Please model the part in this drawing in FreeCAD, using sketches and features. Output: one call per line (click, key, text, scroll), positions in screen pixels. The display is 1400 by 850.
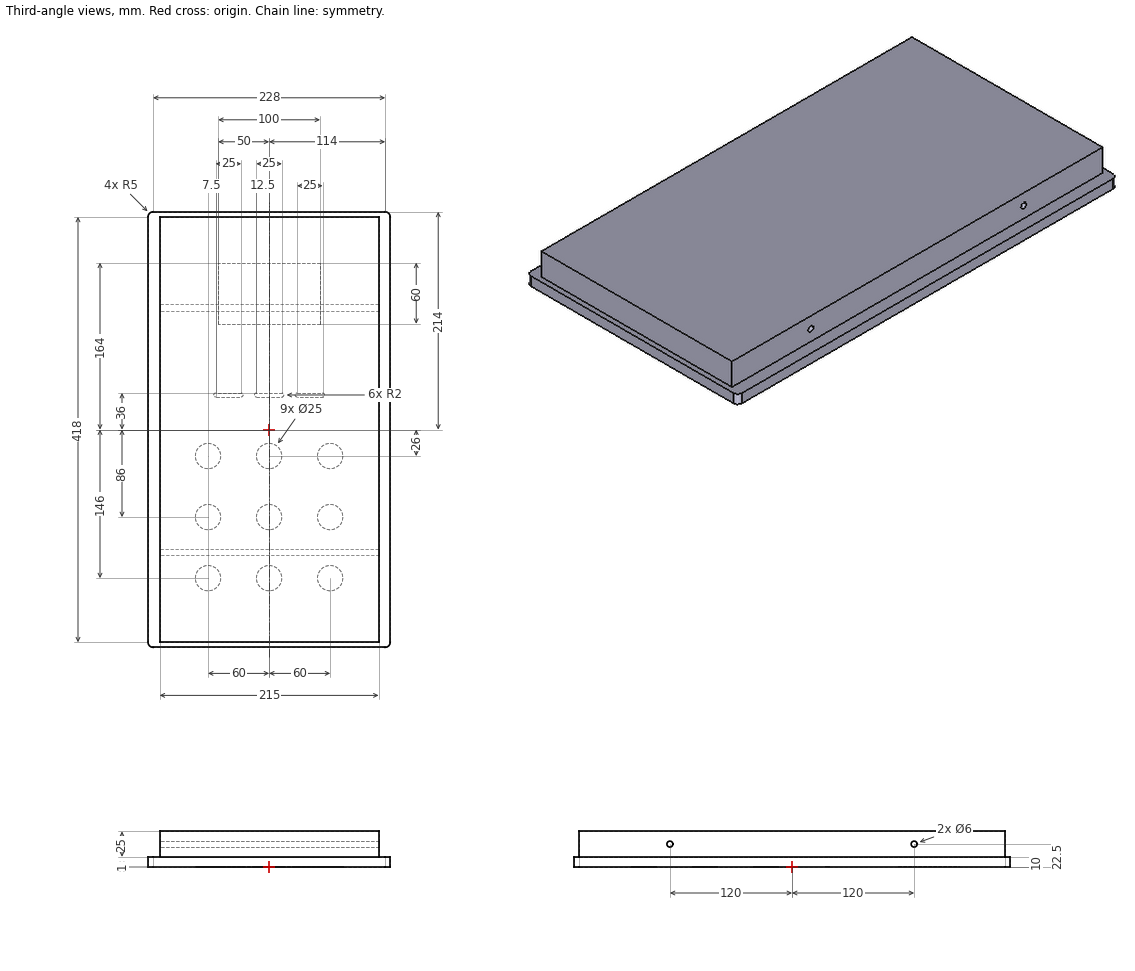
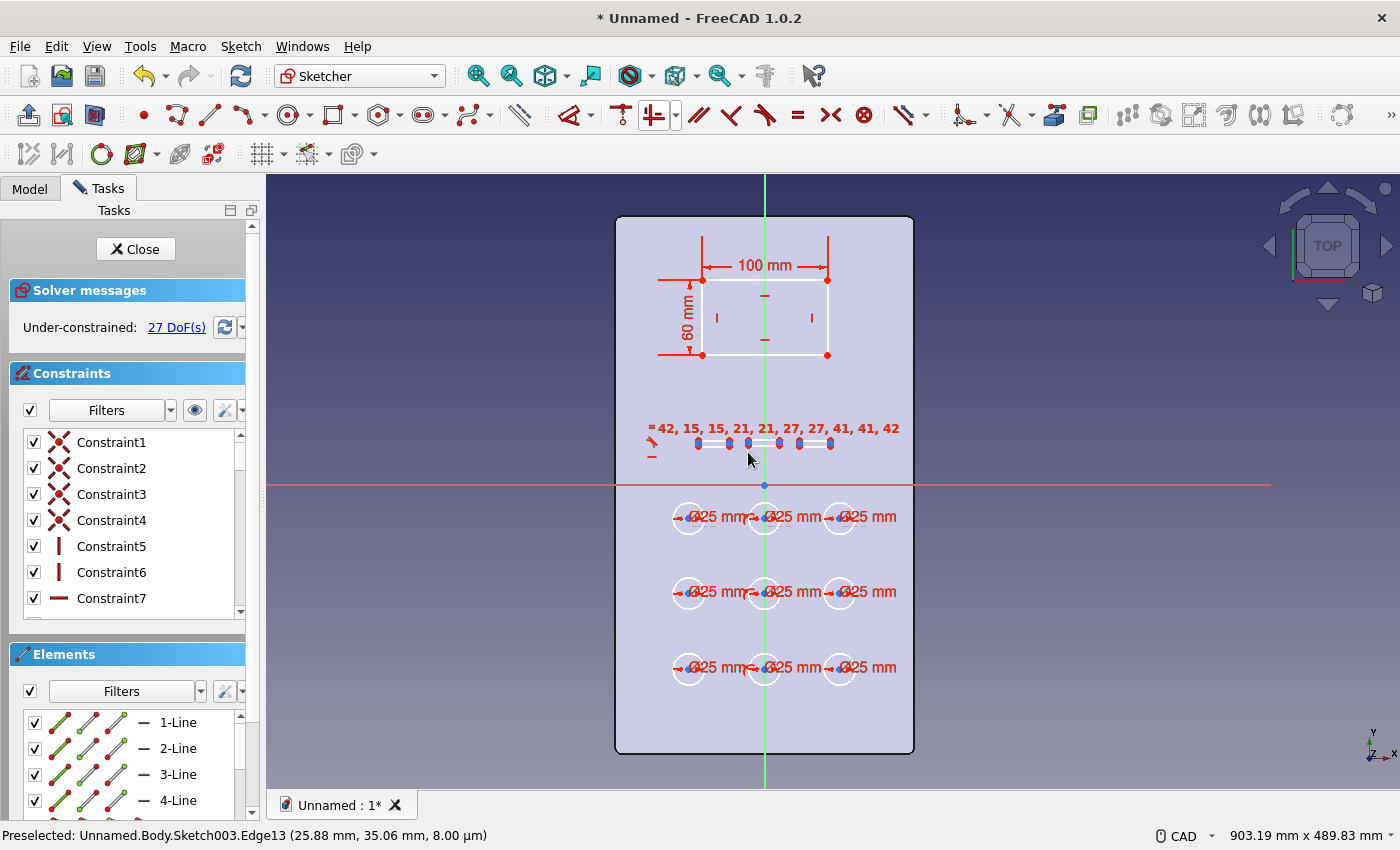
click(765, 519)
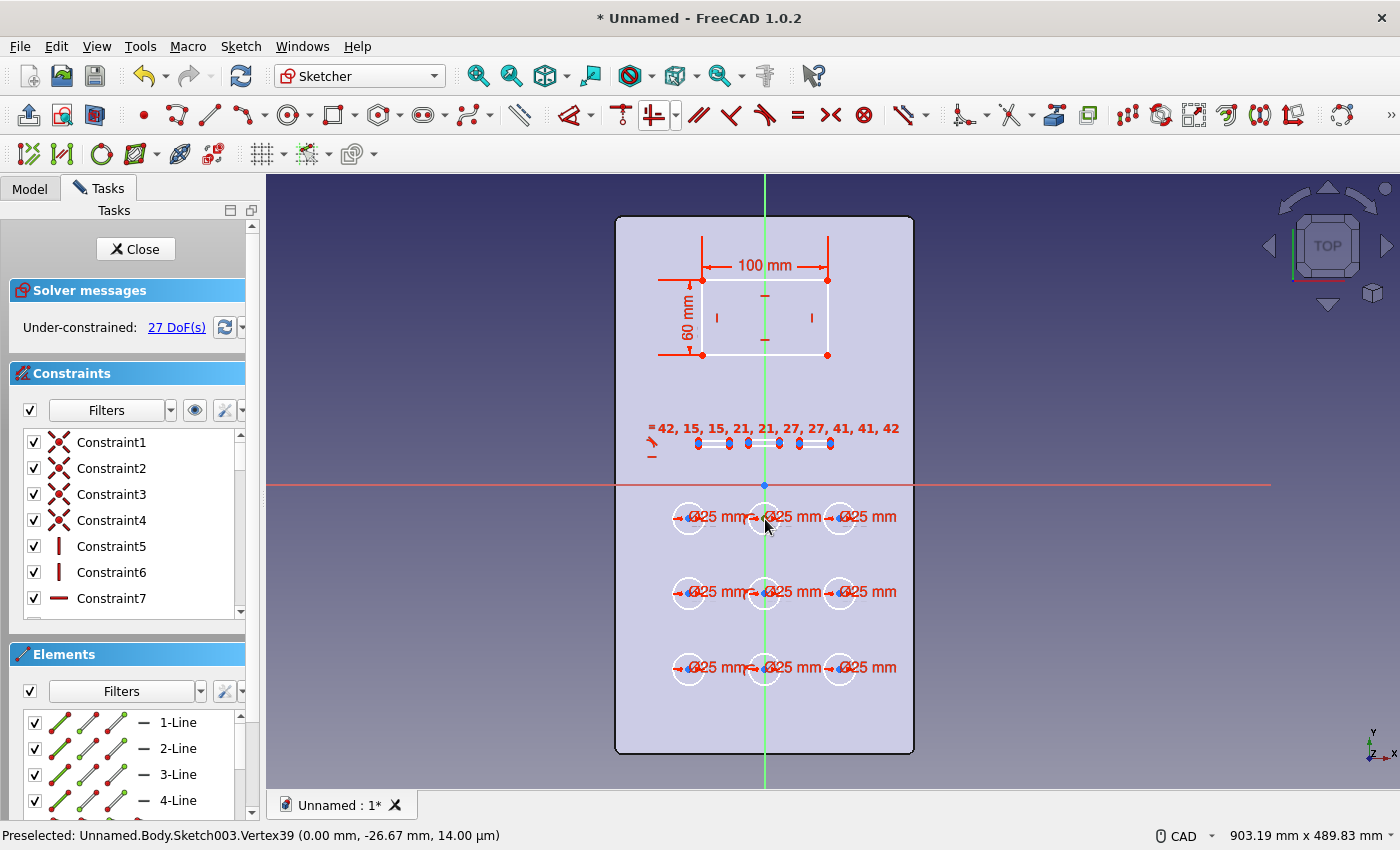
click(689, 519)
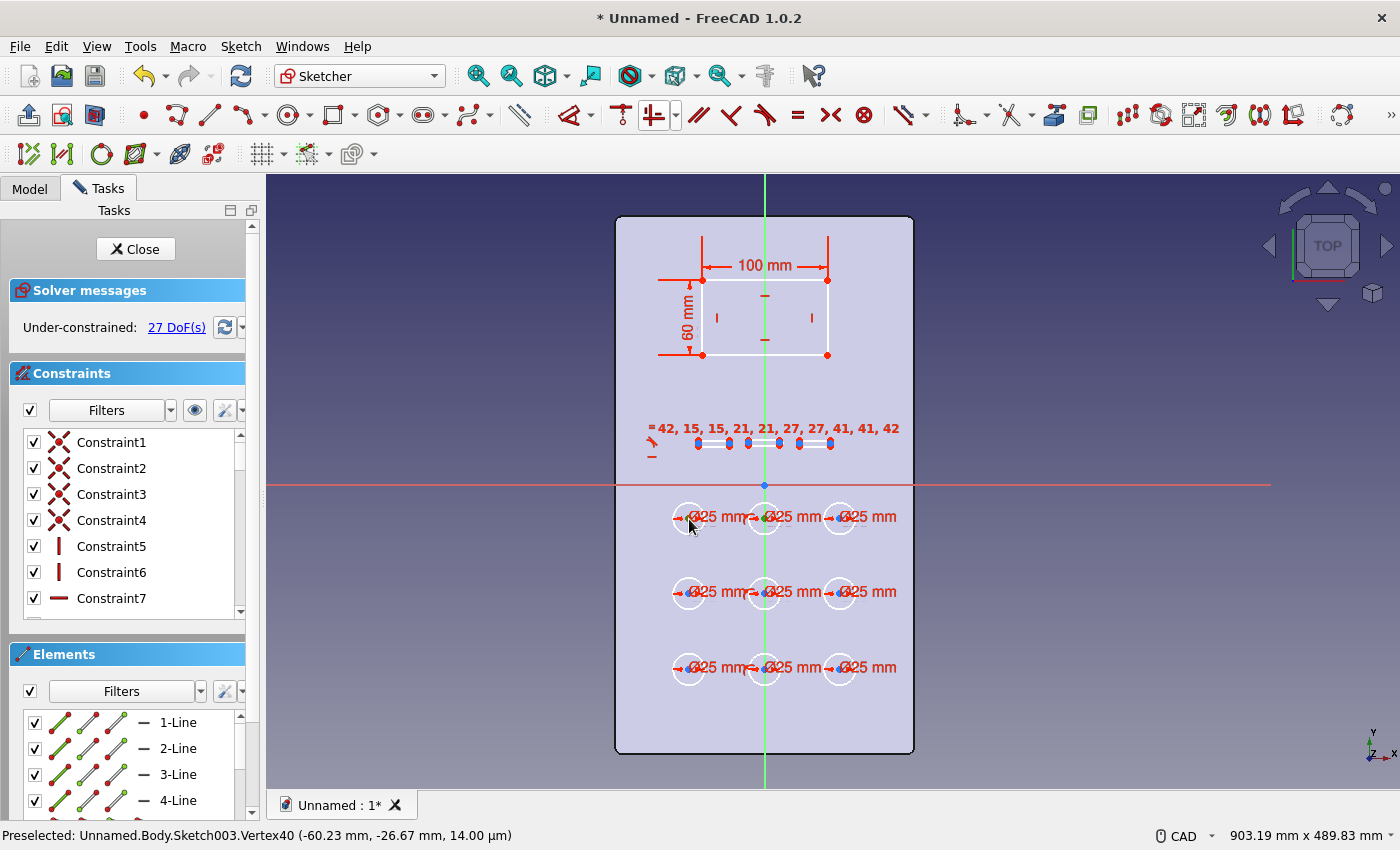
click(676, 116)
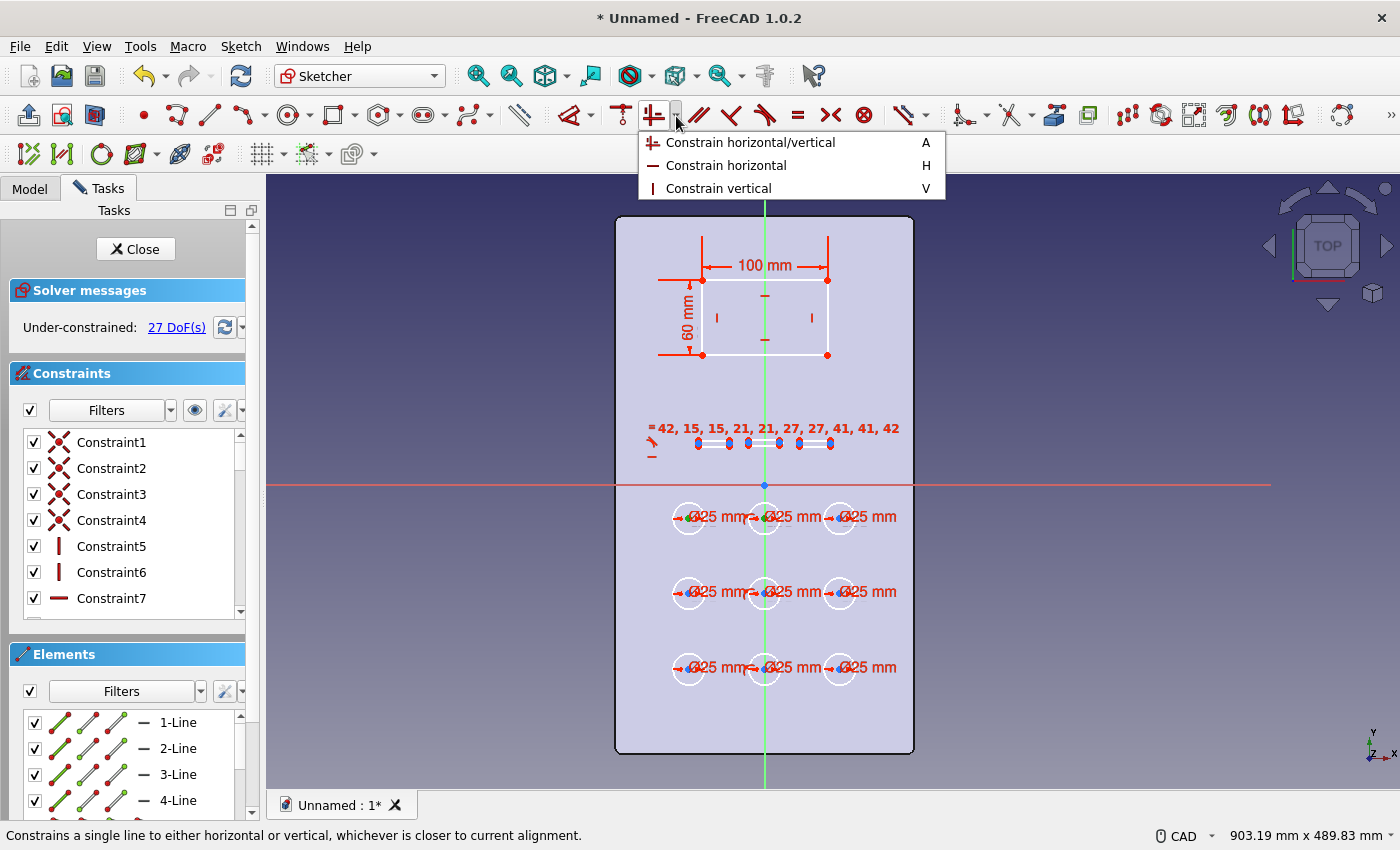
click(792, 166)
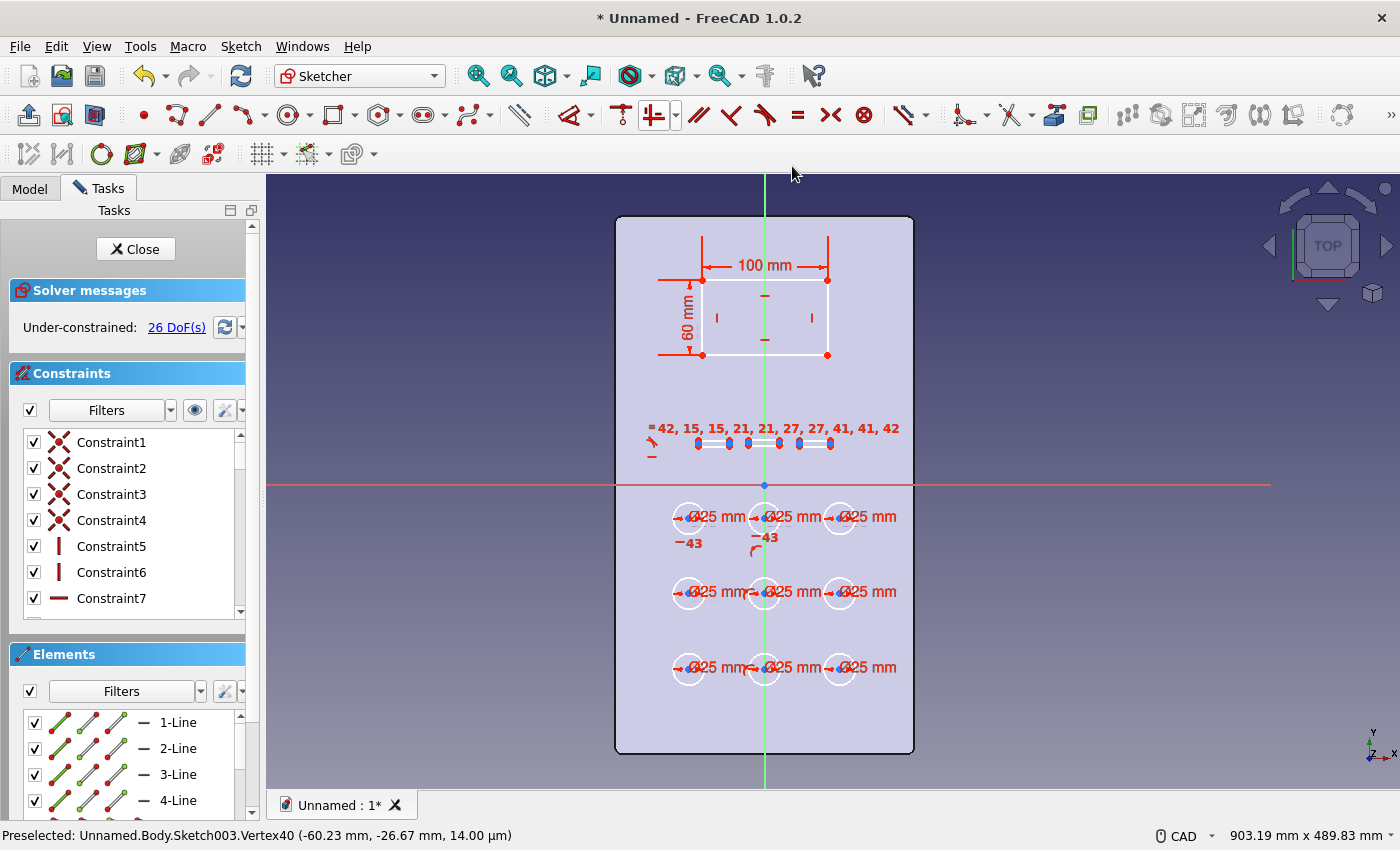
click(689, 519)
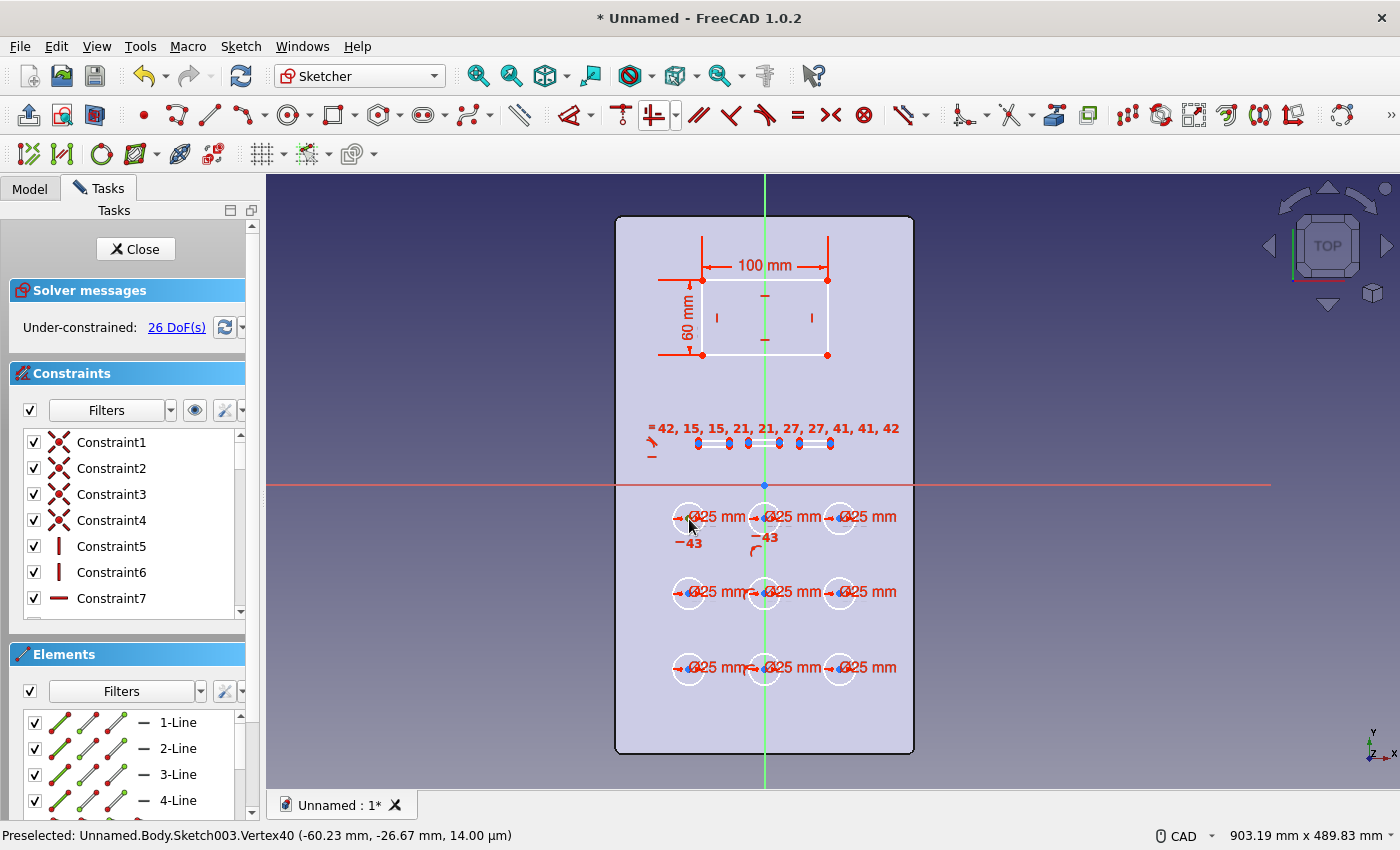
click(689, 594)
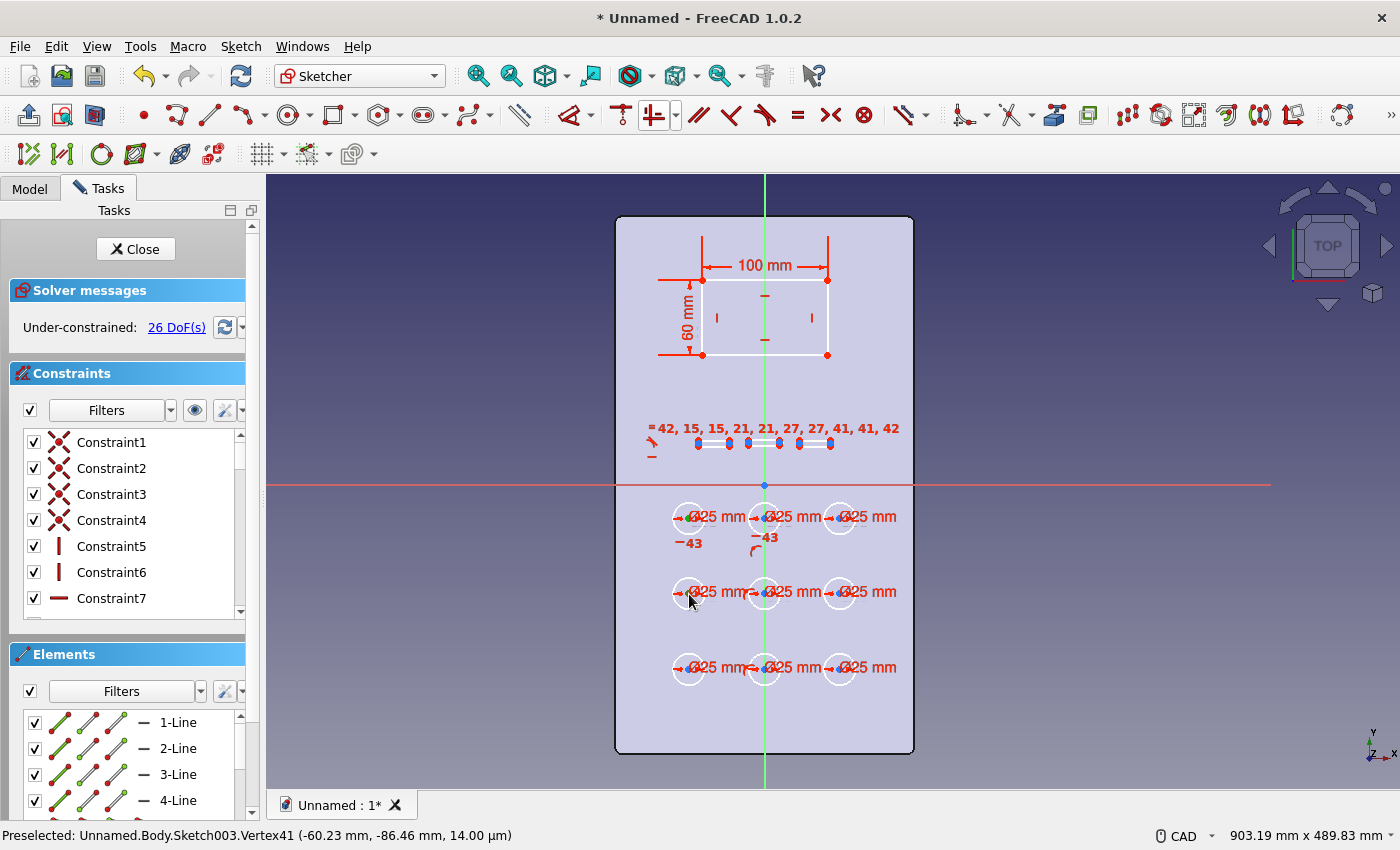
click(676, 116)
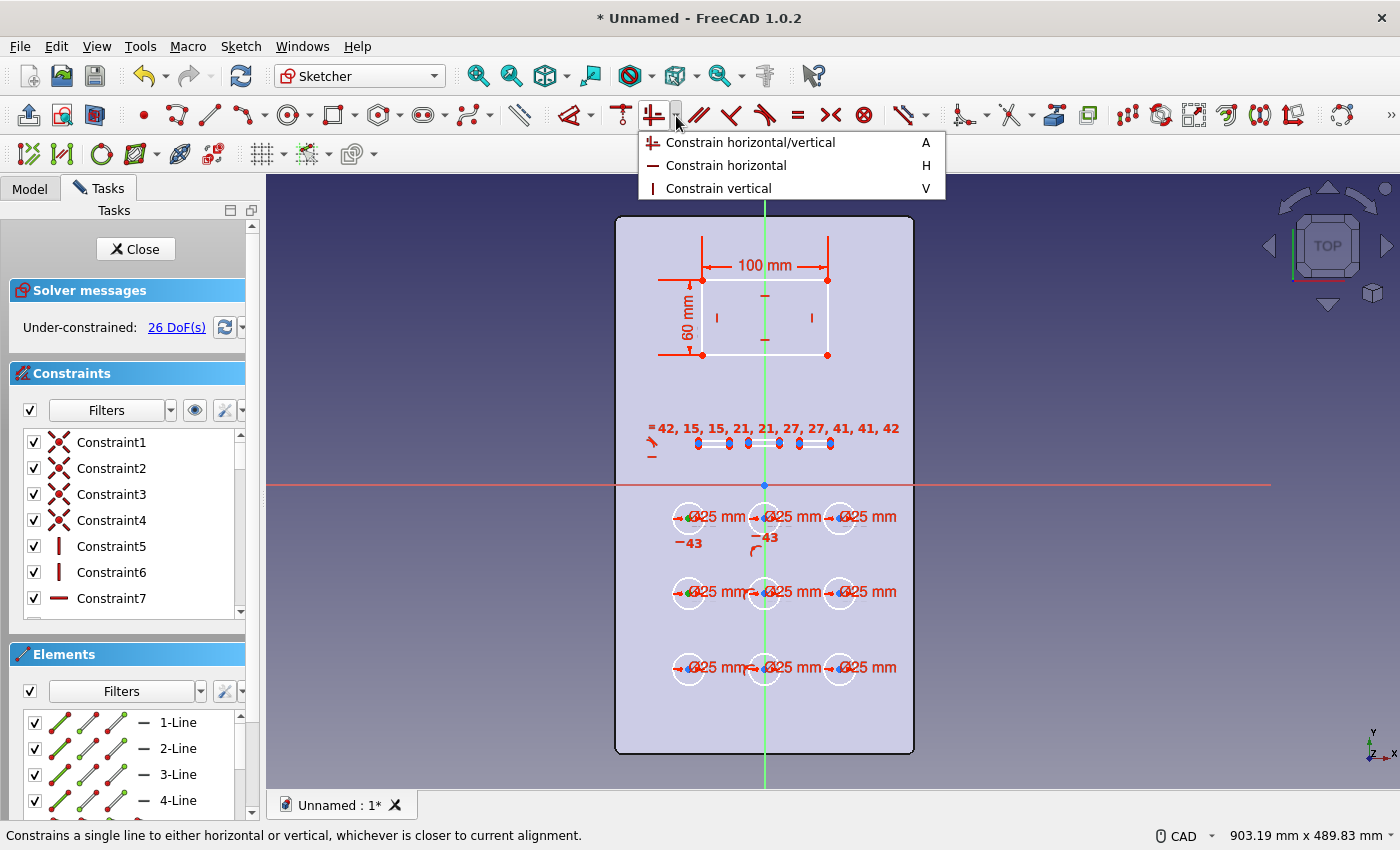
click(792, 188)